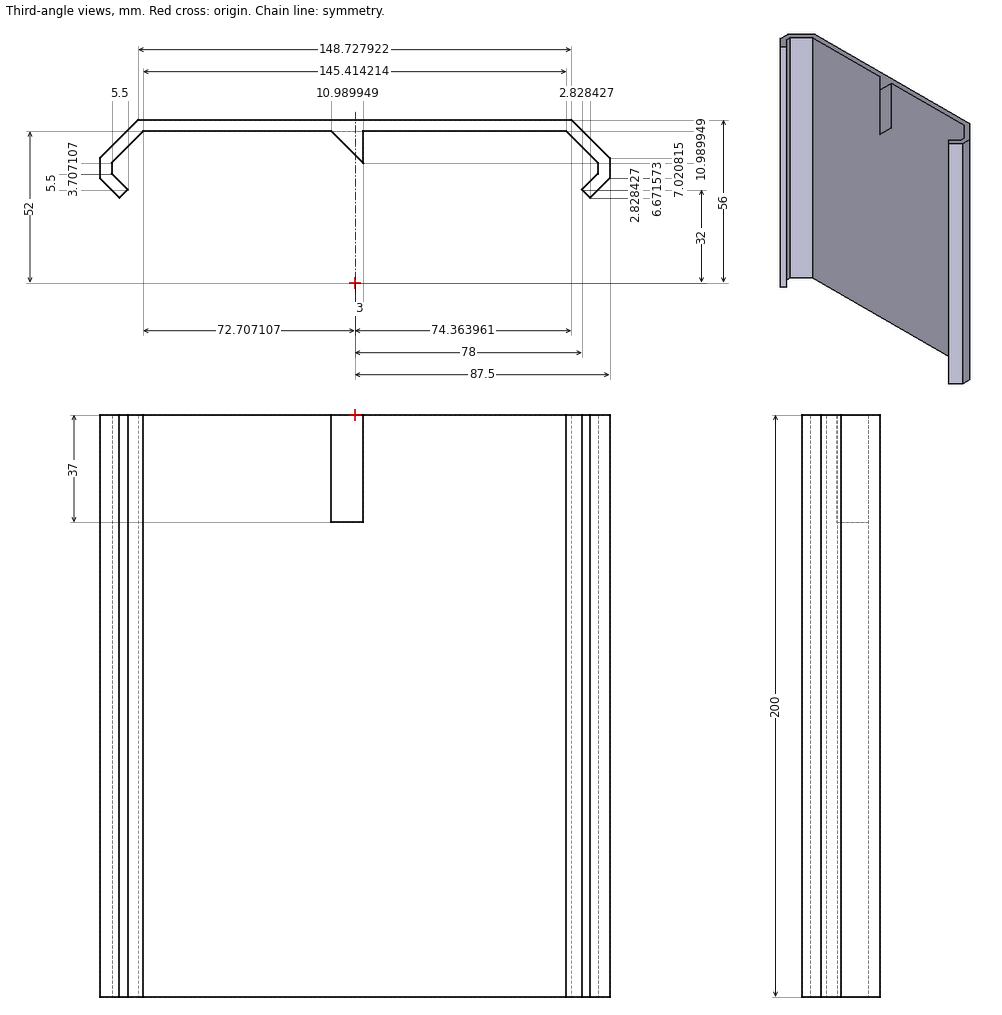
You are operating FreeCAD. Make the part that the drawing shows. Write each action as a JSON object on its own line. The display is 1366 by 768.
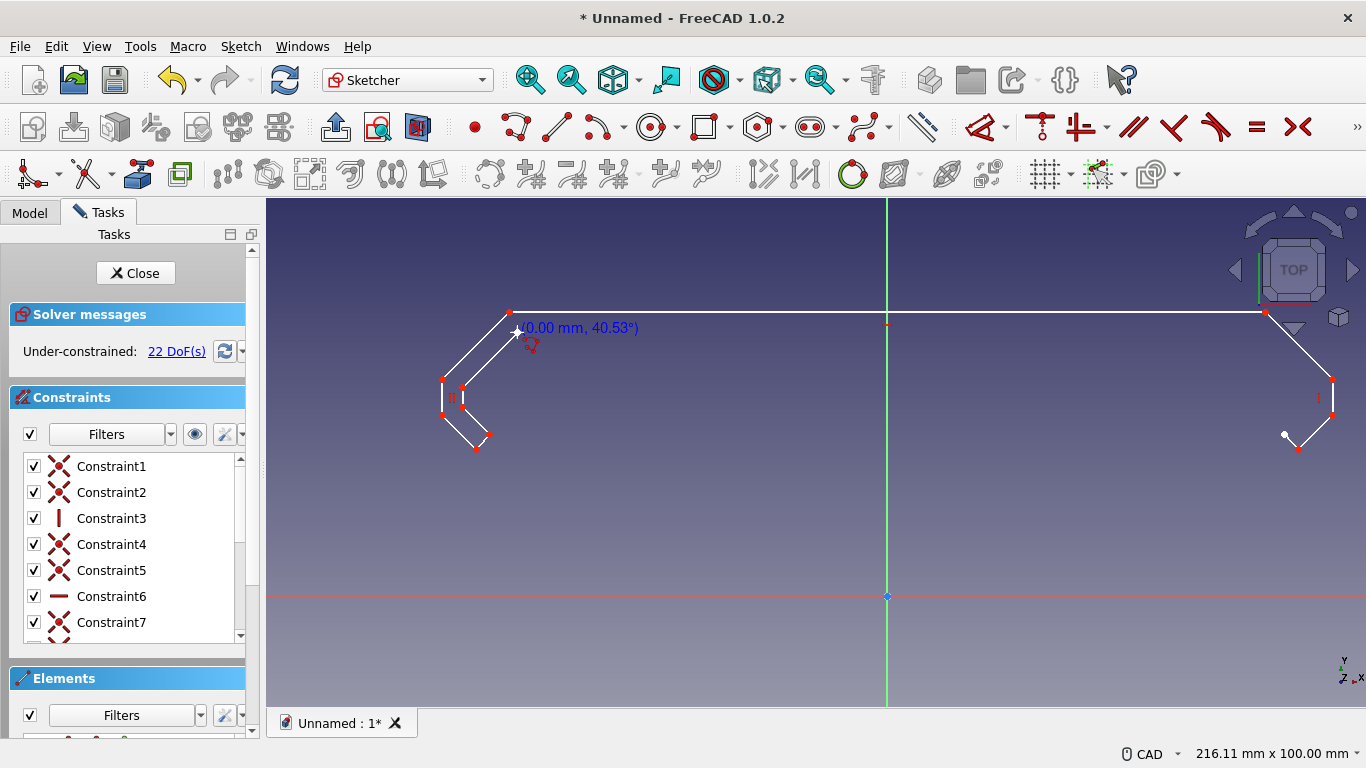
{"action": "scroll", "coordinate": [463, 450], "scroll_direction": "down", "scroll_amount": 2}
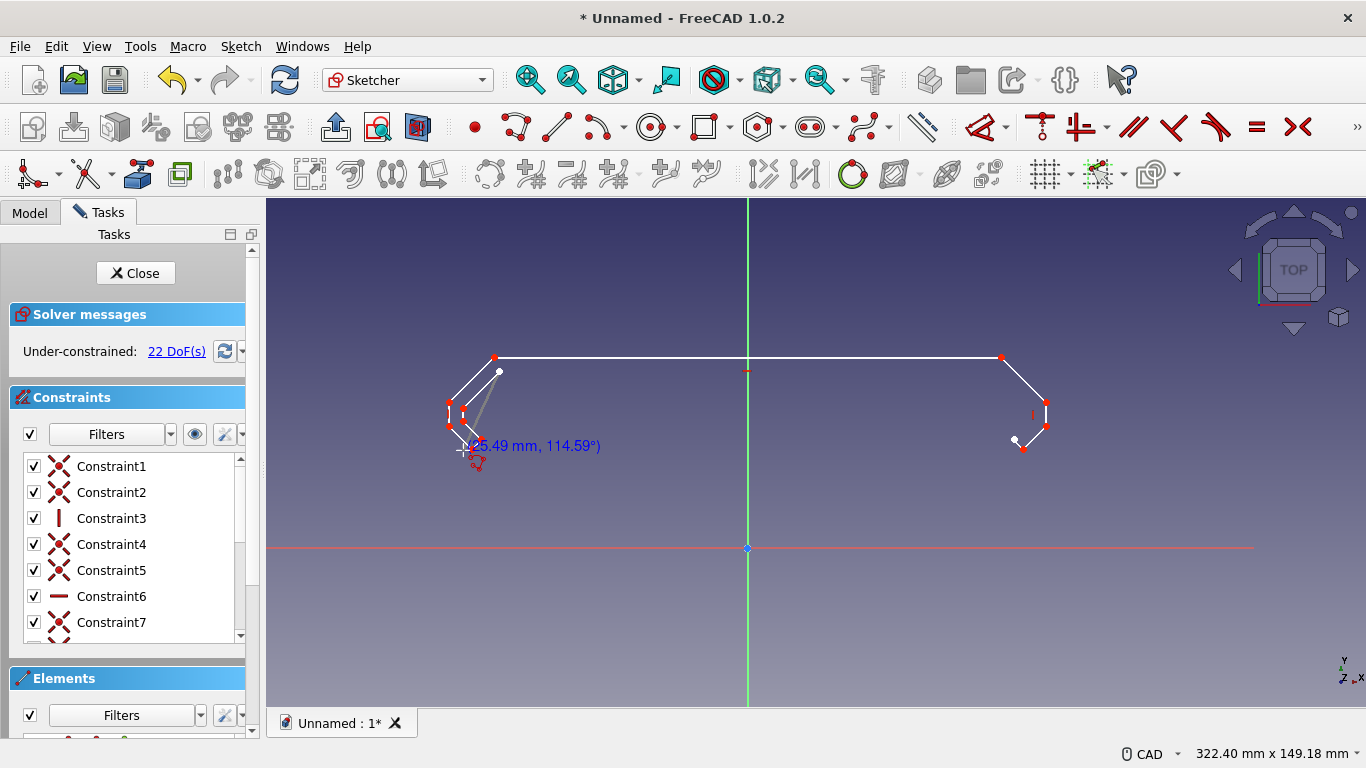
{"action": "left_click", "coordinate": [996, 371]}
{"action": "left_click", "coordinate": [1032, 408]}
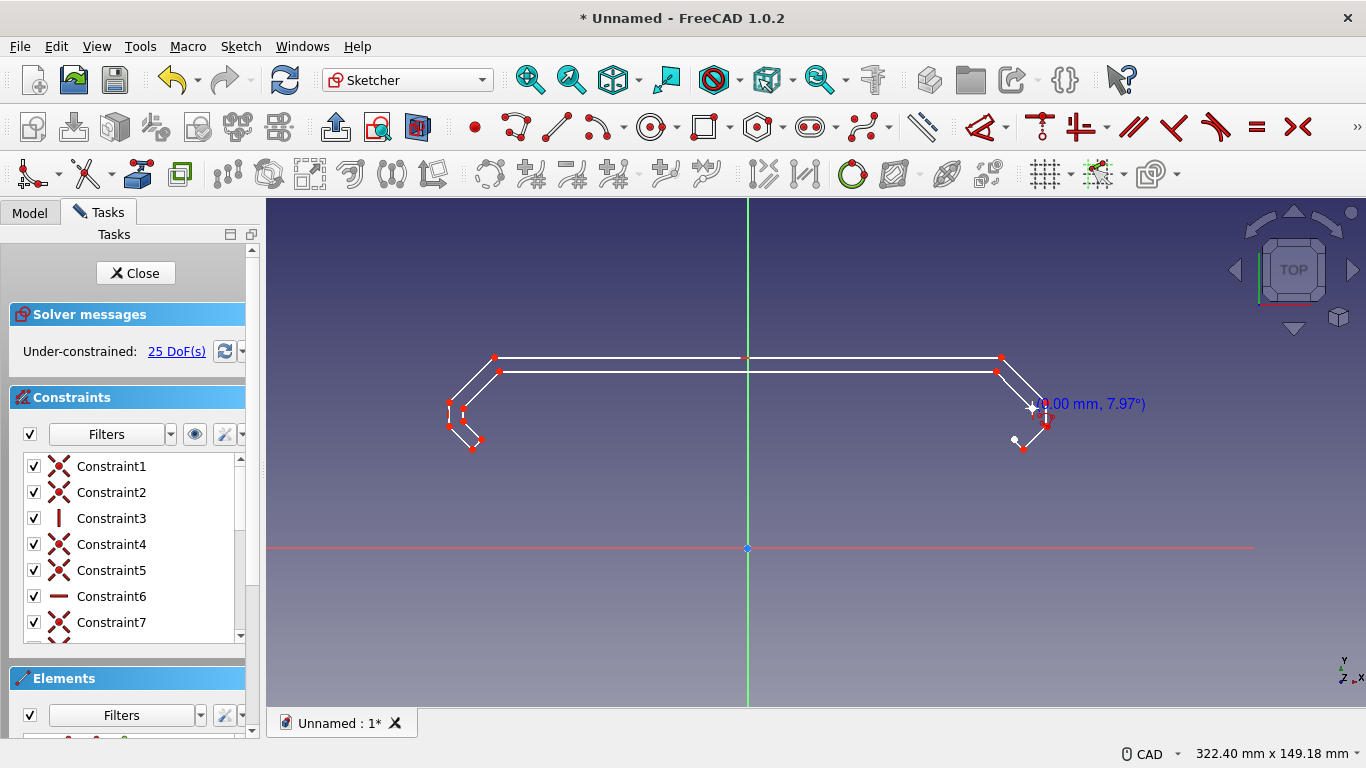
{"action": "scroll", "coordinate": [1032, 420], "scroll_direction": "up", "scroll_amount": 2}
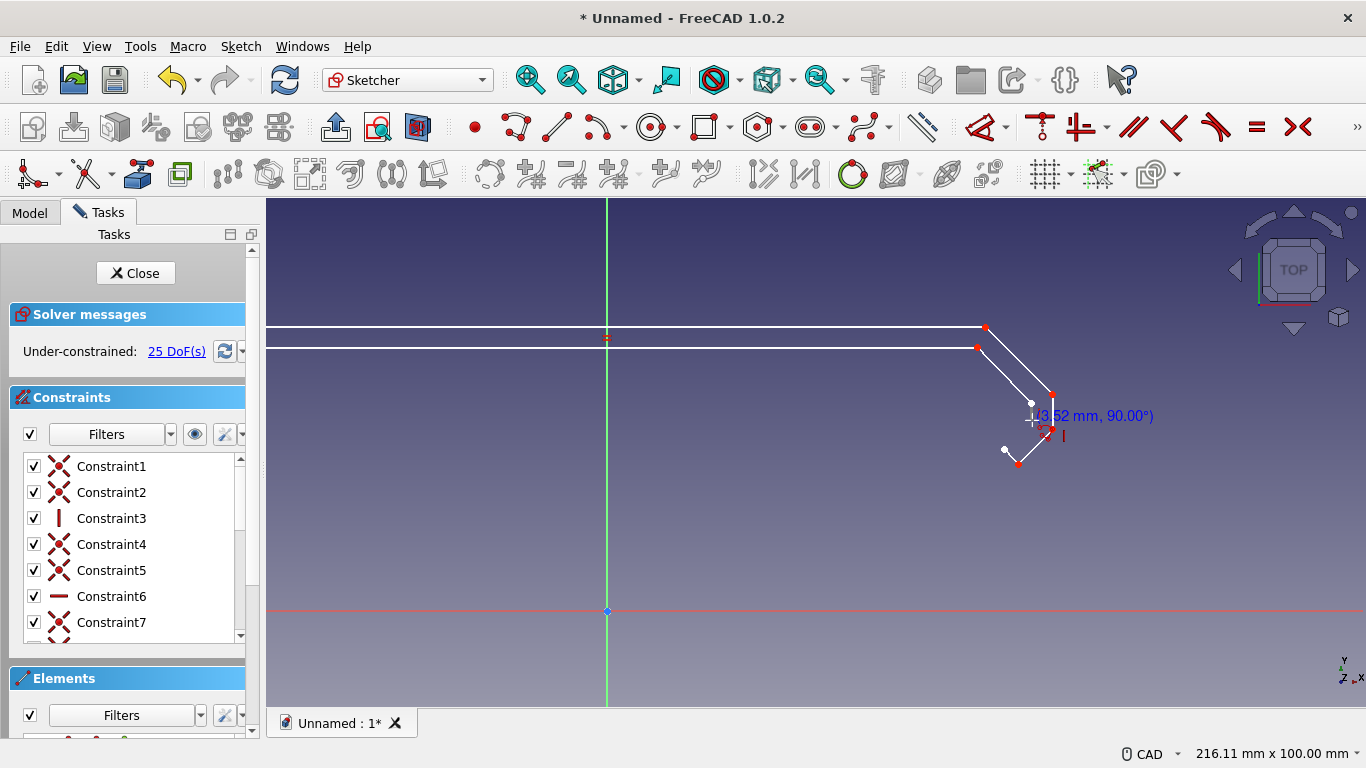
{"action": "left_click", "coordinate": [1032, 420]}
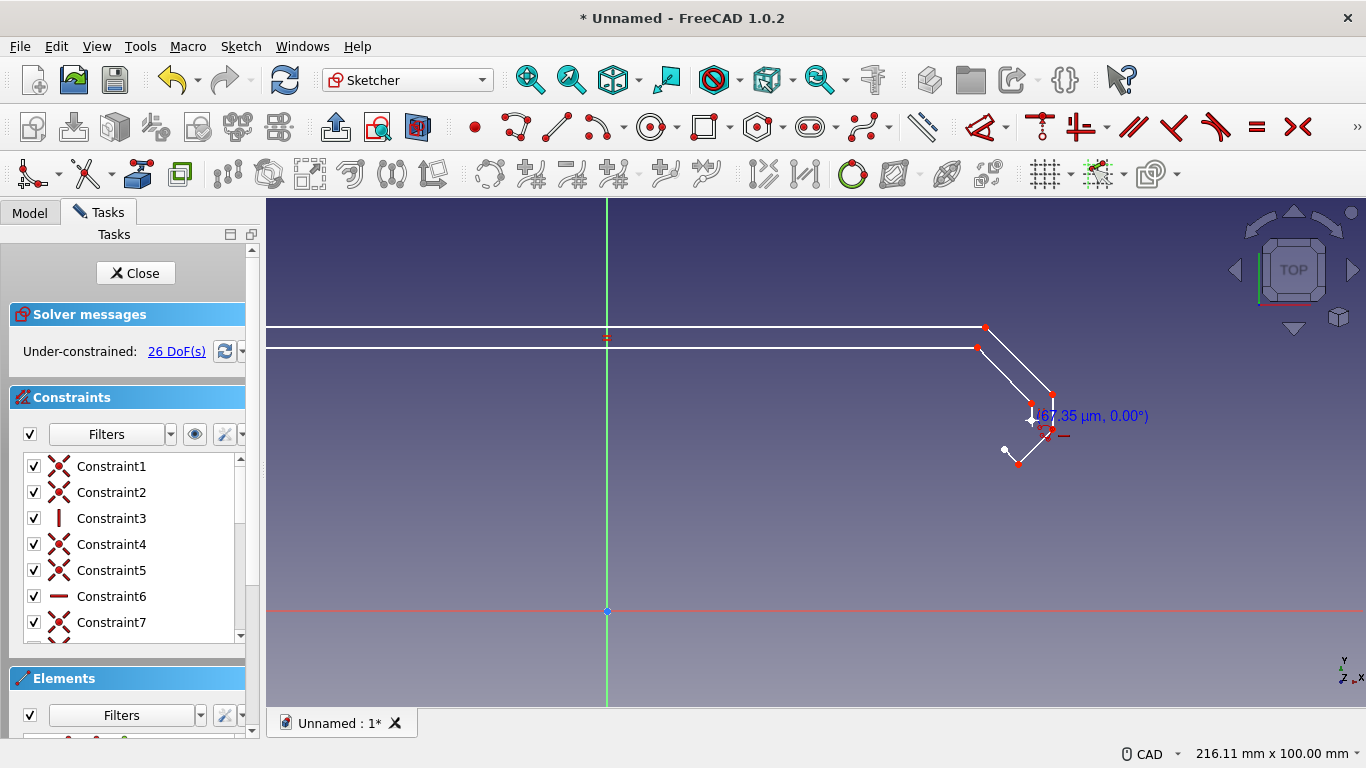
{"action": "scroll", "coordinate": [1004, 448], "scroll_direction": "up", "scroll_amount": 3}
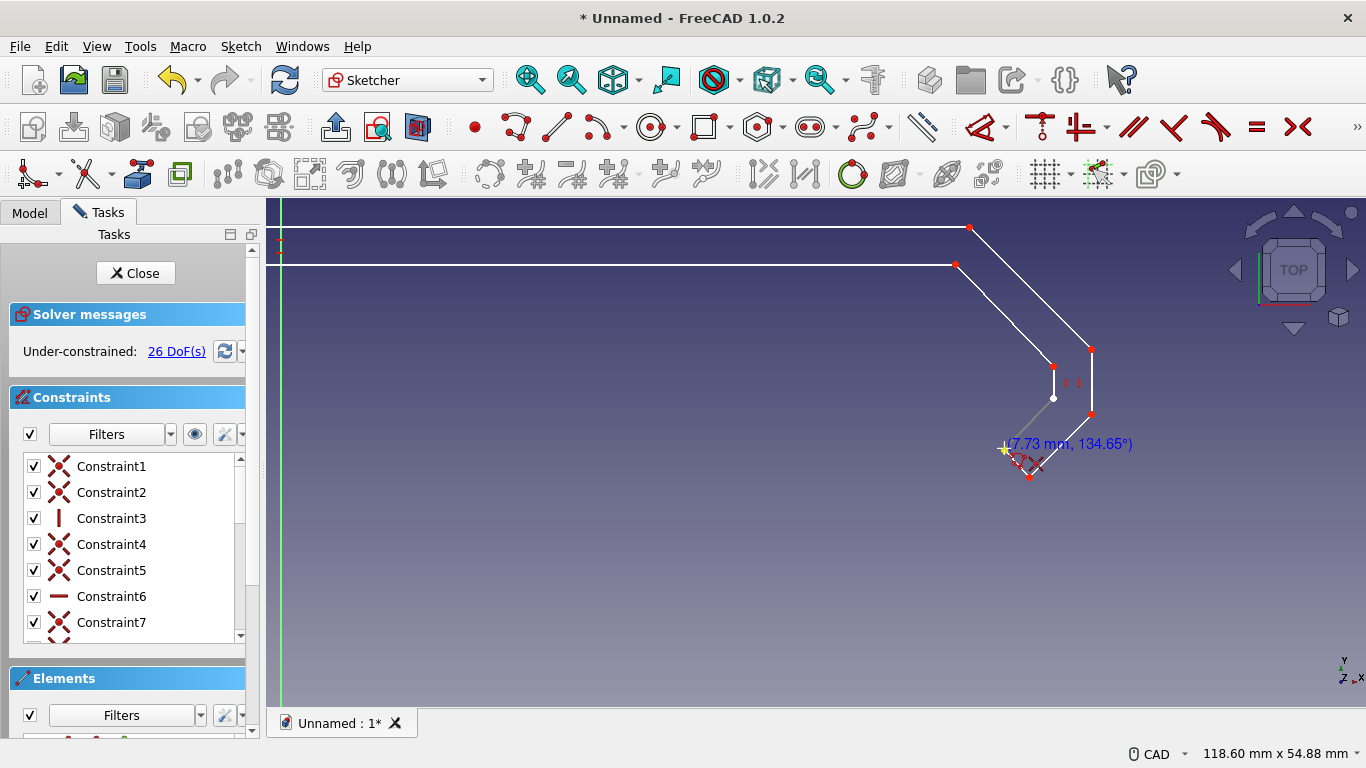
{"action": "left_click", "coordinate": [1005, 450]}
{"action": "key", "text": "Escape"}
{"action": "key", "text": "Escape"}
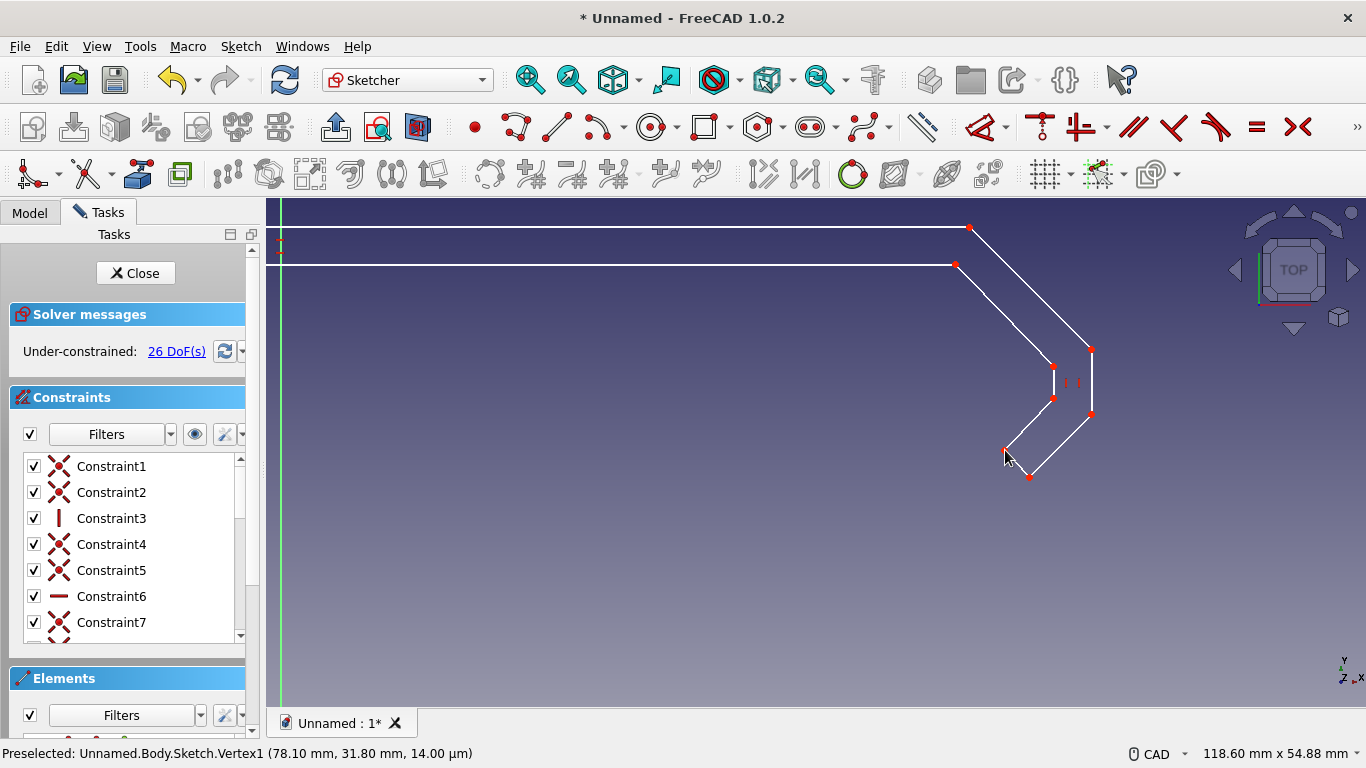
{"action": "left_click", "coordinate": [1092, 349]}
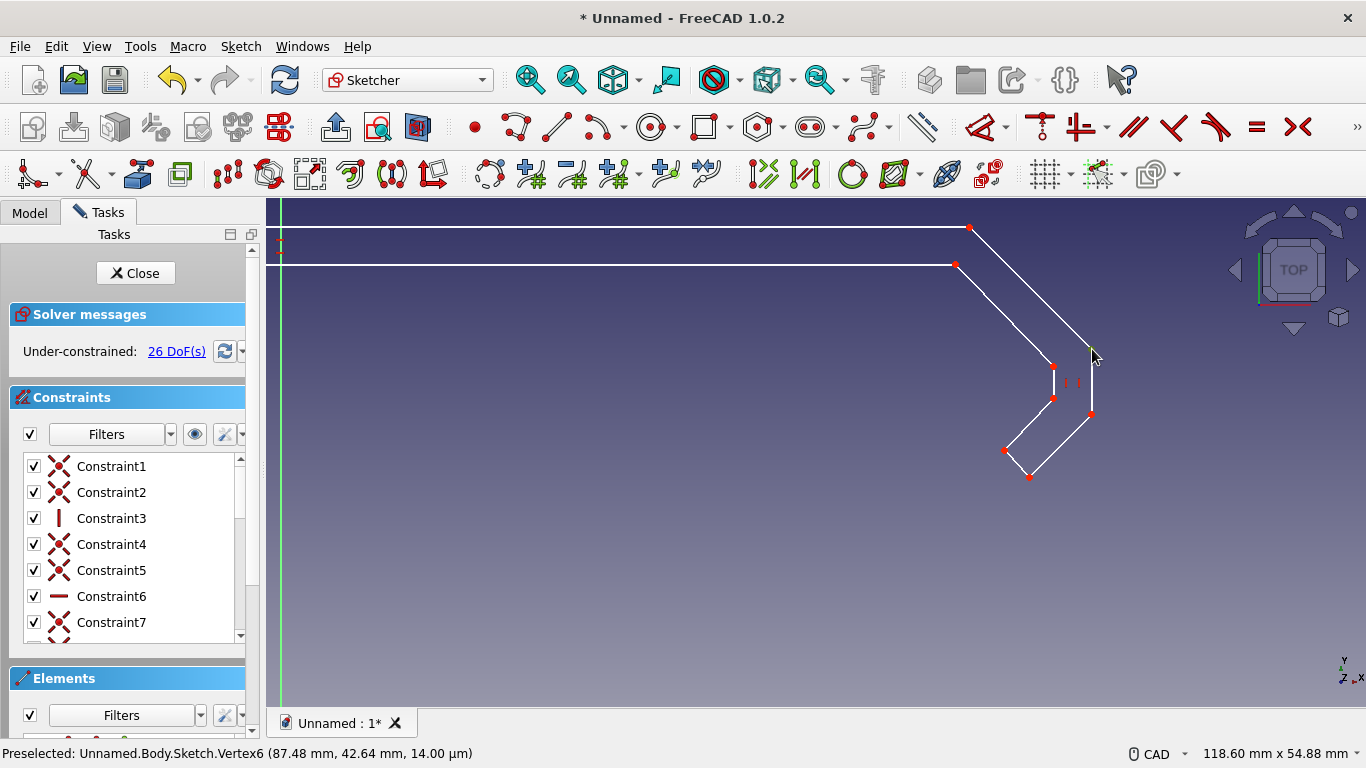
{"action": "scroll", "coordinate": [1019, 433], "scroll_direction": "down", "scroll_amount": 5}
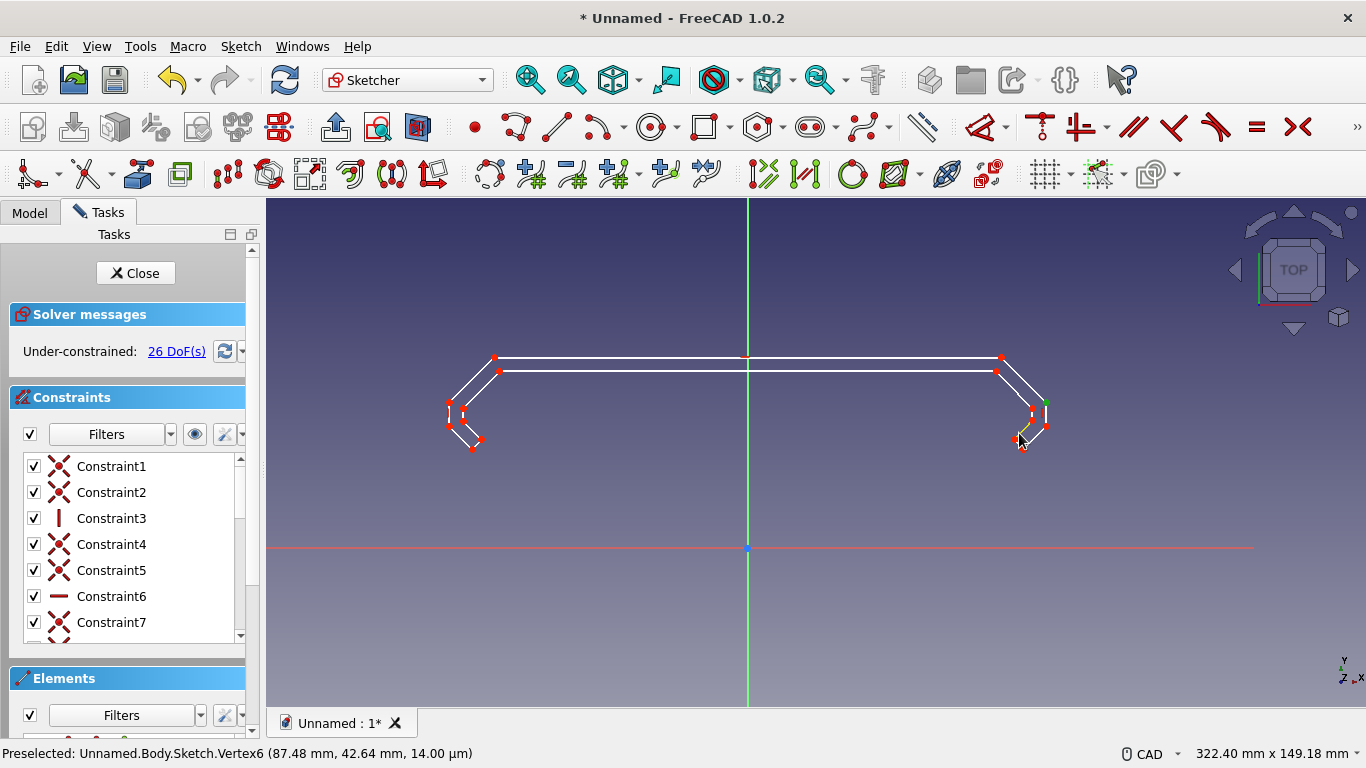
{"action": "left_click", "coordinate": [449, 403]}